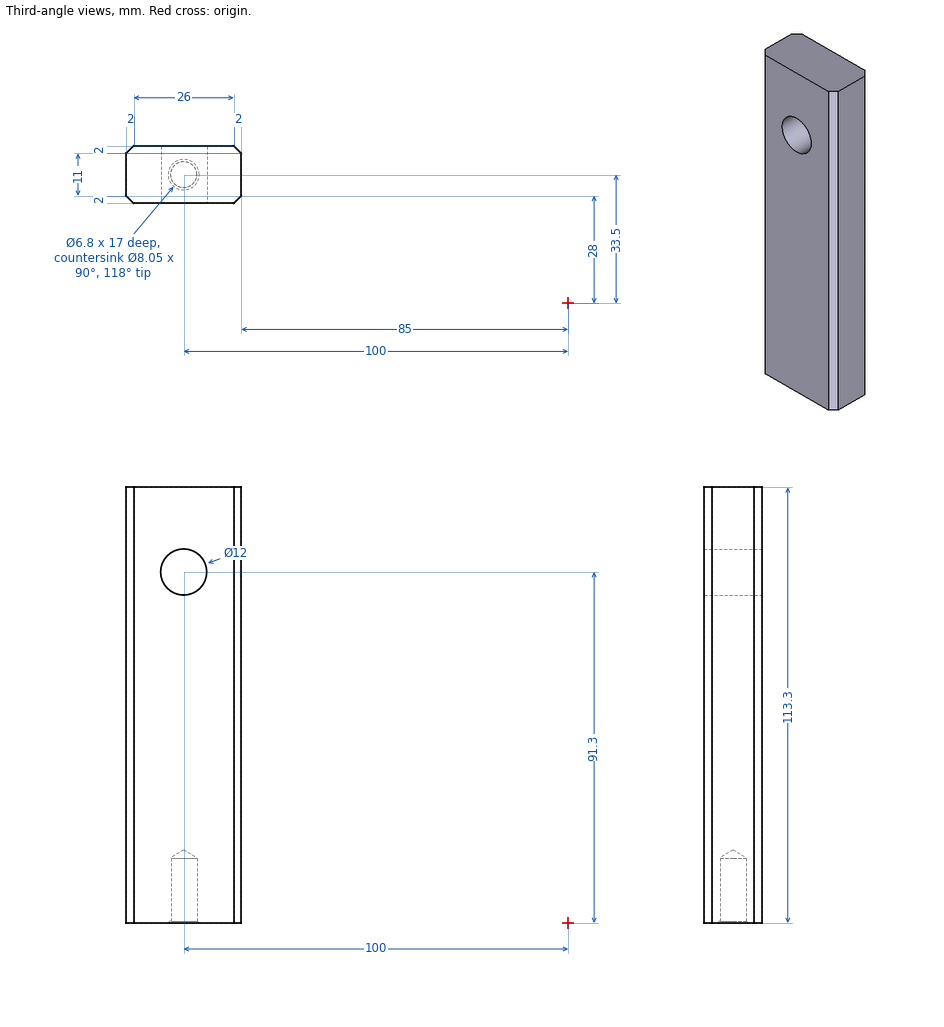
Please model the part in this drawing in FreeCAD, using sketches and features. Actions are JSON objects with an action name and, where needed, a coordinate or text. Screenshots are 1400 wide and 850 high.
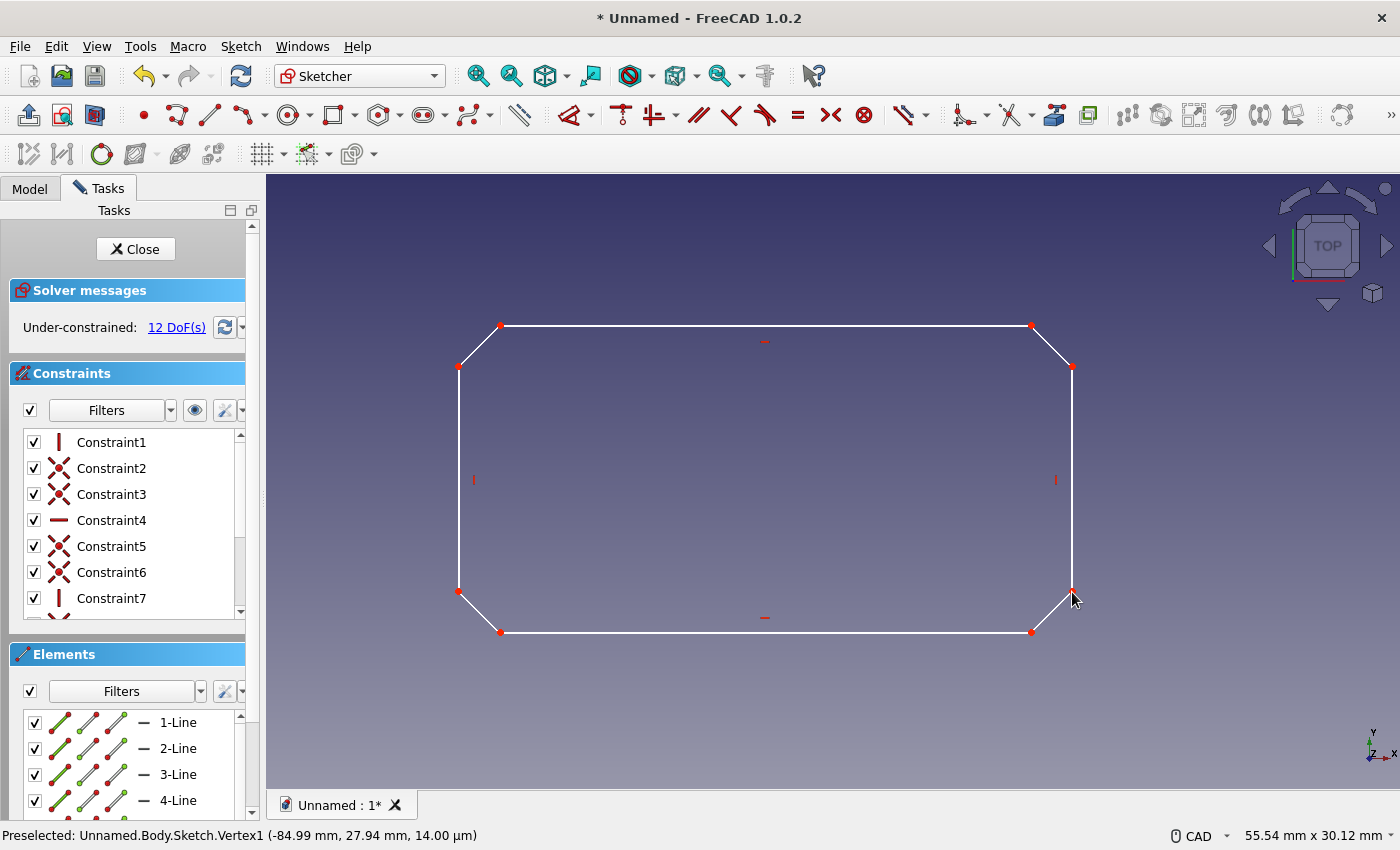
{"action": "left_click", "coordinate": [1072, 524]}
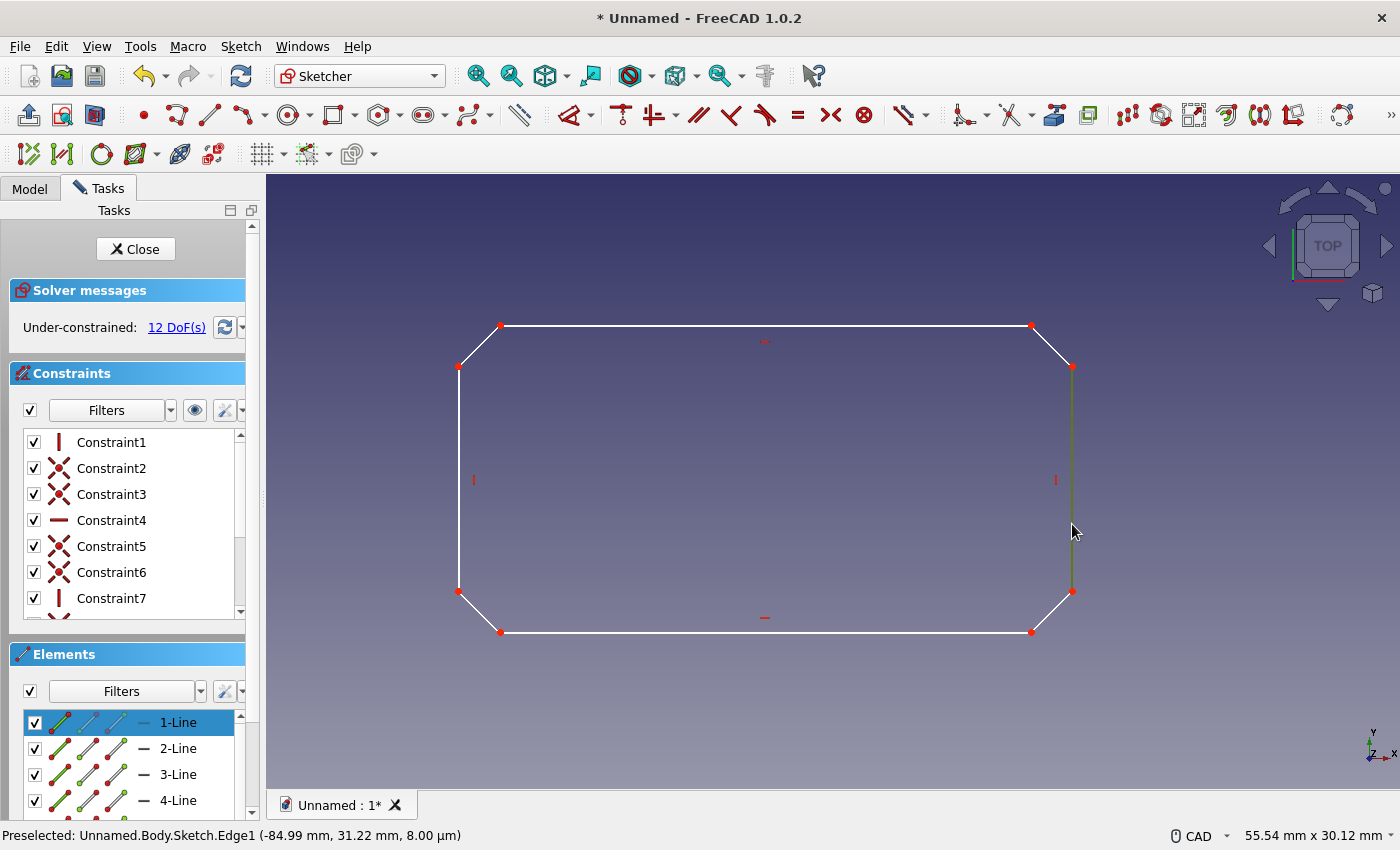
{"action": "left_click", "coordinate": [590, 116]}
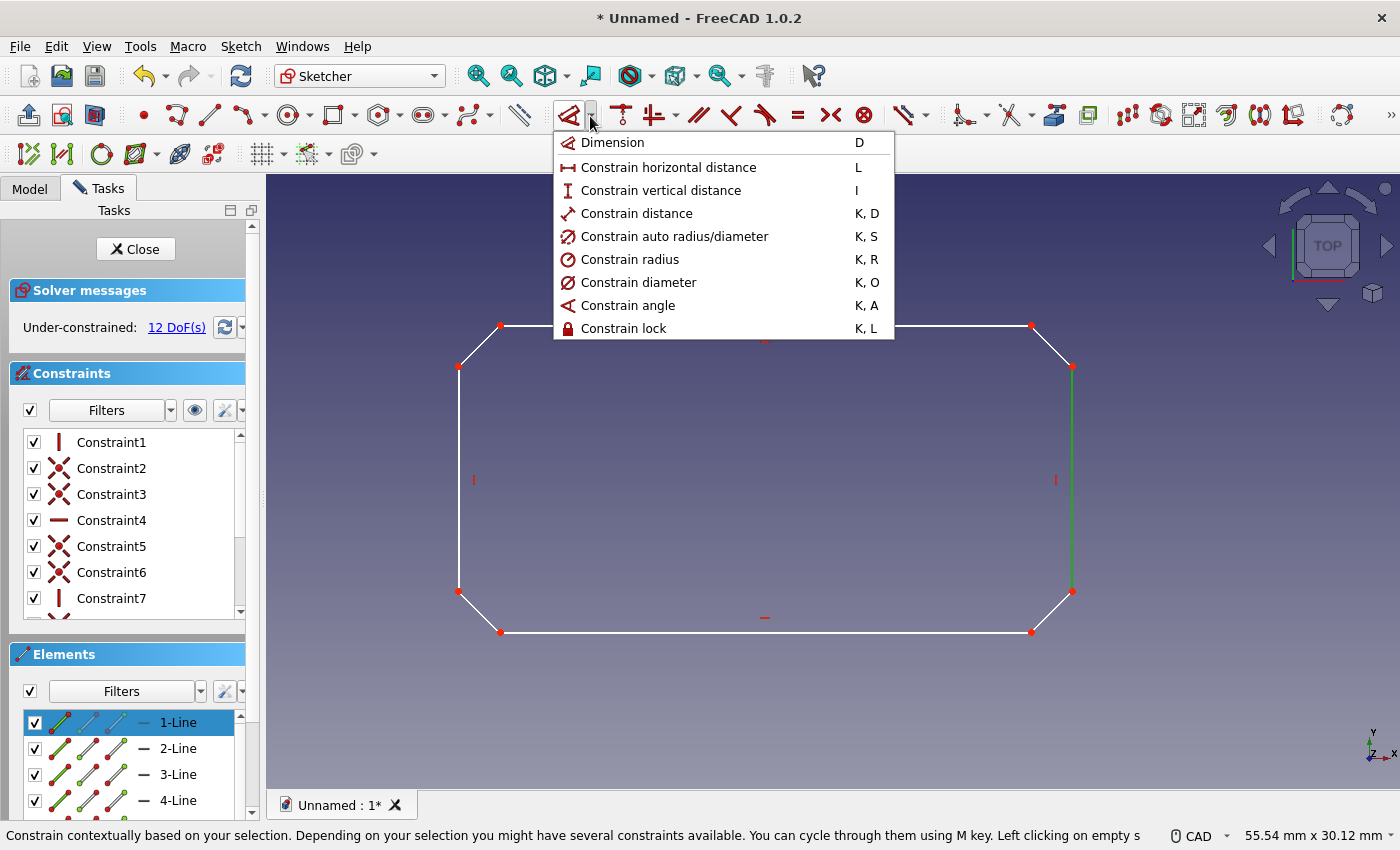
{"action": "left_click", "coordinate": [724, 190]}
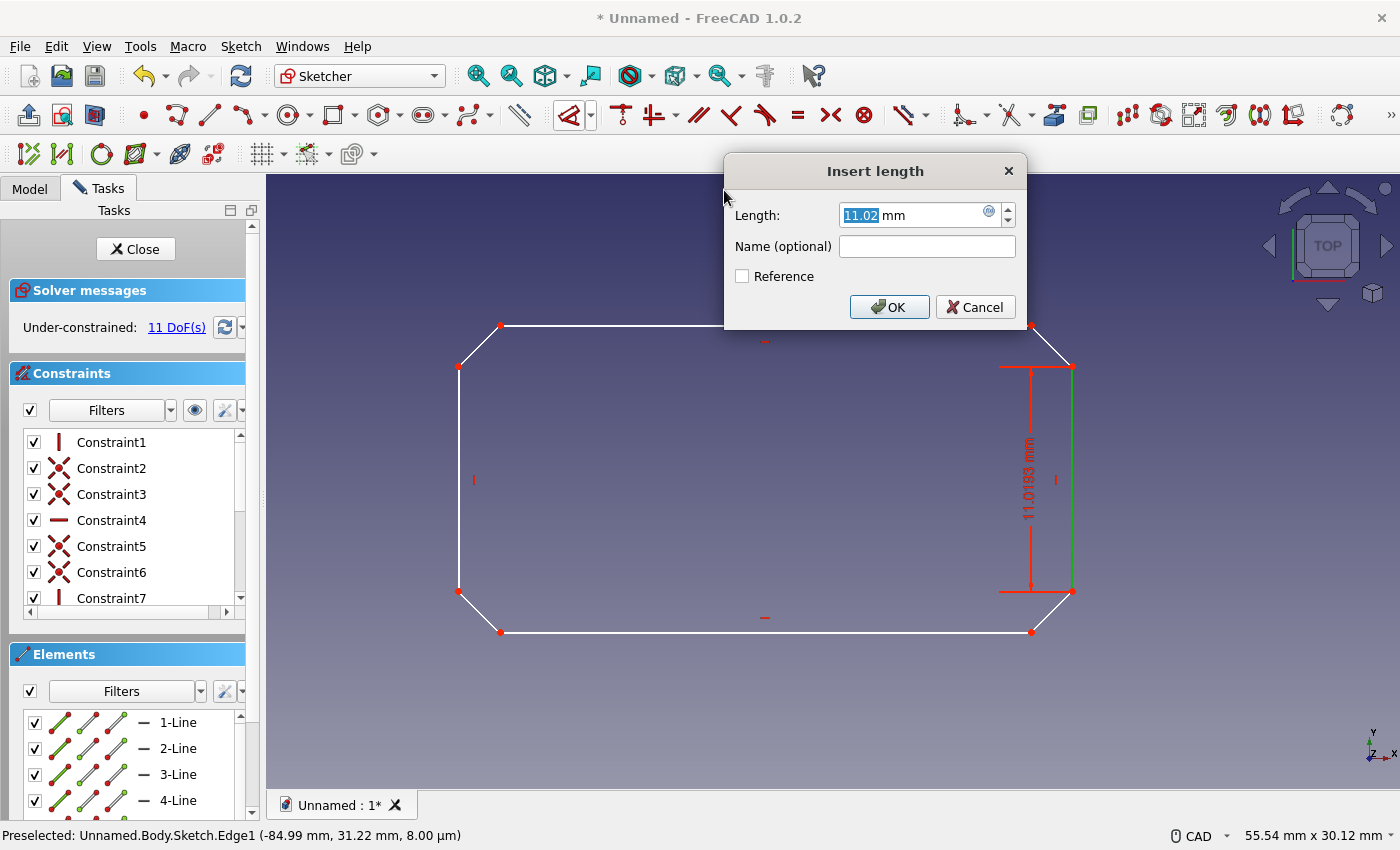
{"action": "type", "text": "11"}
{"action": "key", "text": "Return"}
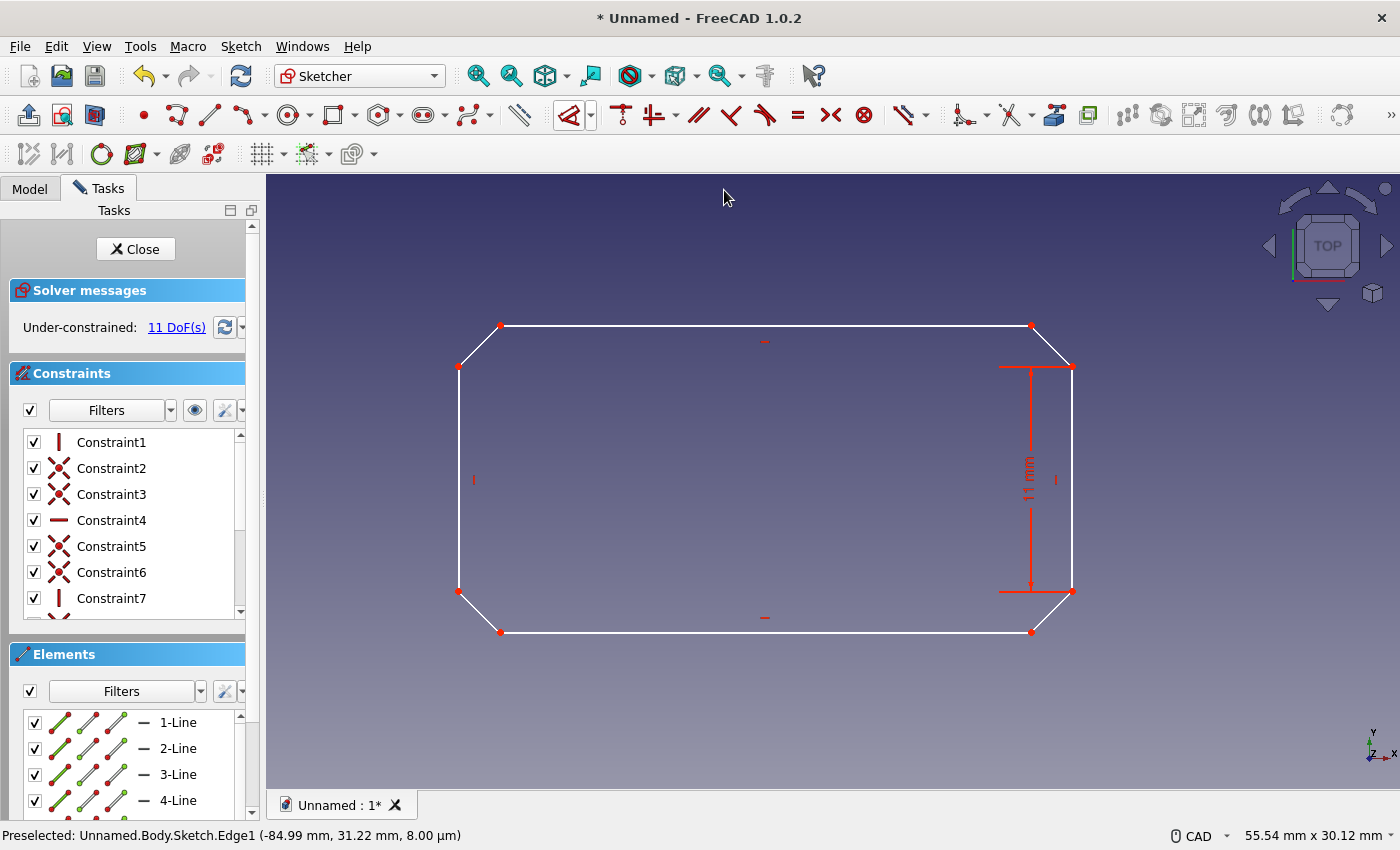
{"action": "left_click", "coordinate": [872, 326]}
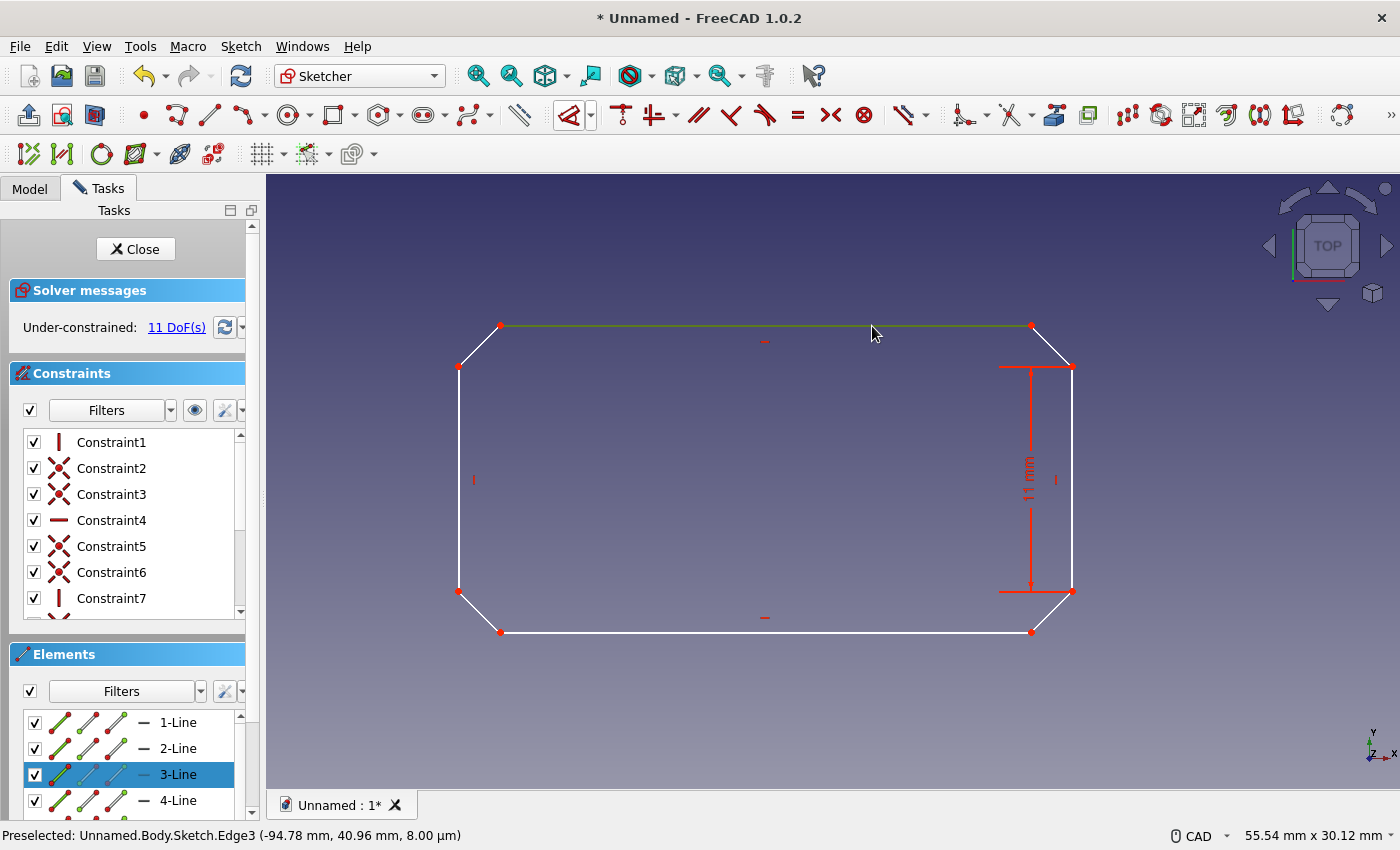
{"action": "left_click", "coordinate": [590, 116]}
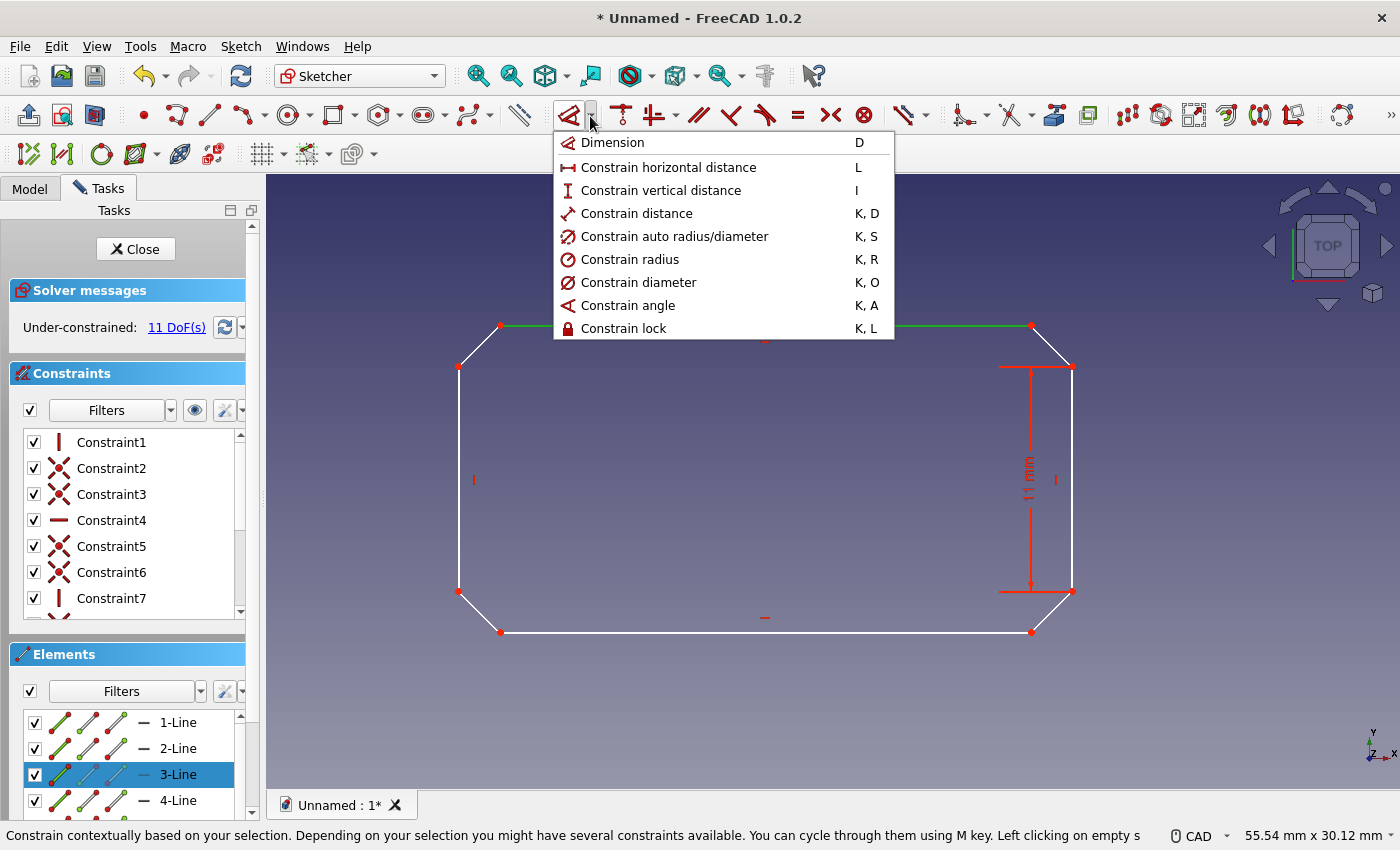
{"action": "left_click", "coordinate": [724, 168]}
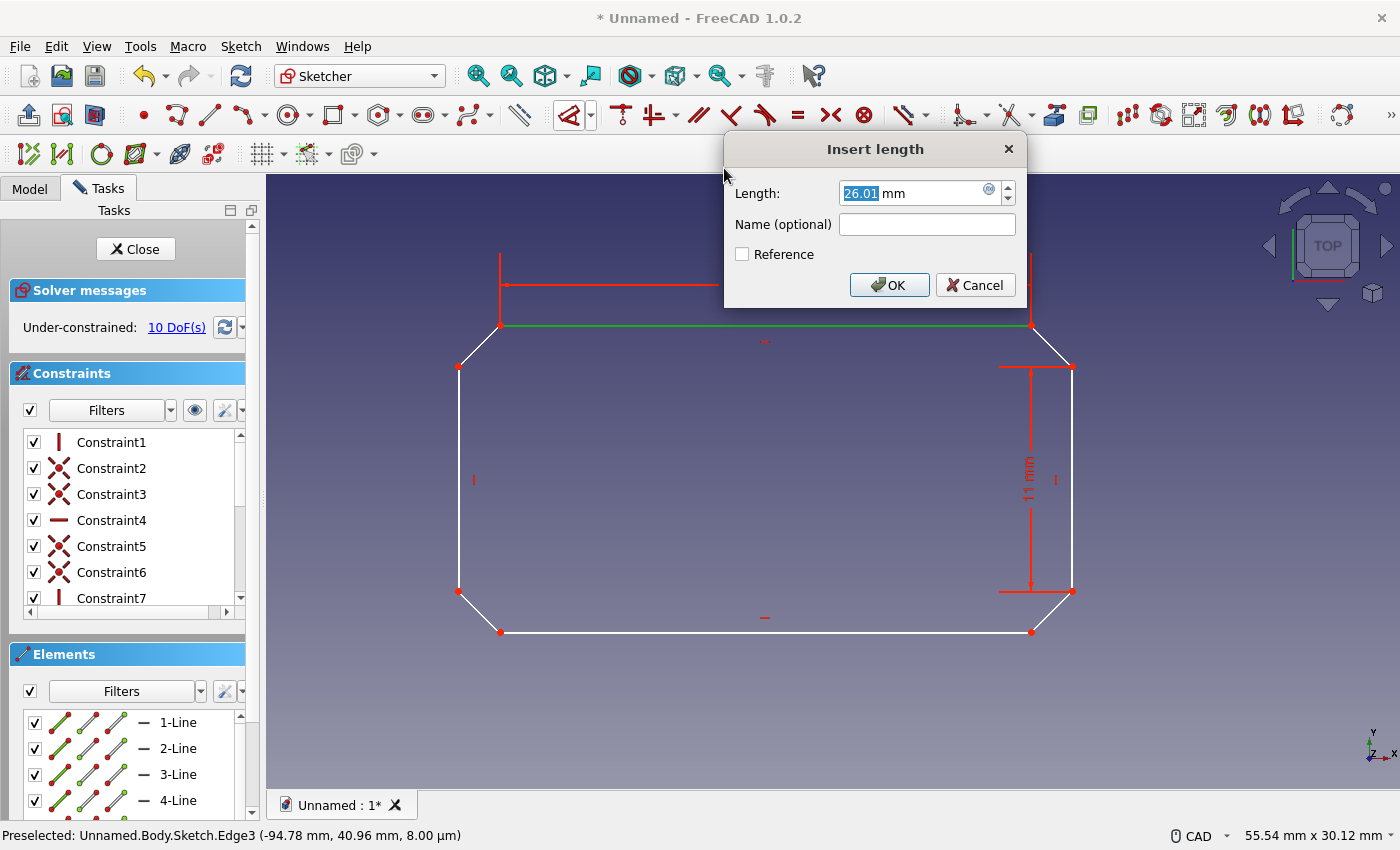
{"action": "type", "text": "26"}
{"action": "key", "text": "Return"}